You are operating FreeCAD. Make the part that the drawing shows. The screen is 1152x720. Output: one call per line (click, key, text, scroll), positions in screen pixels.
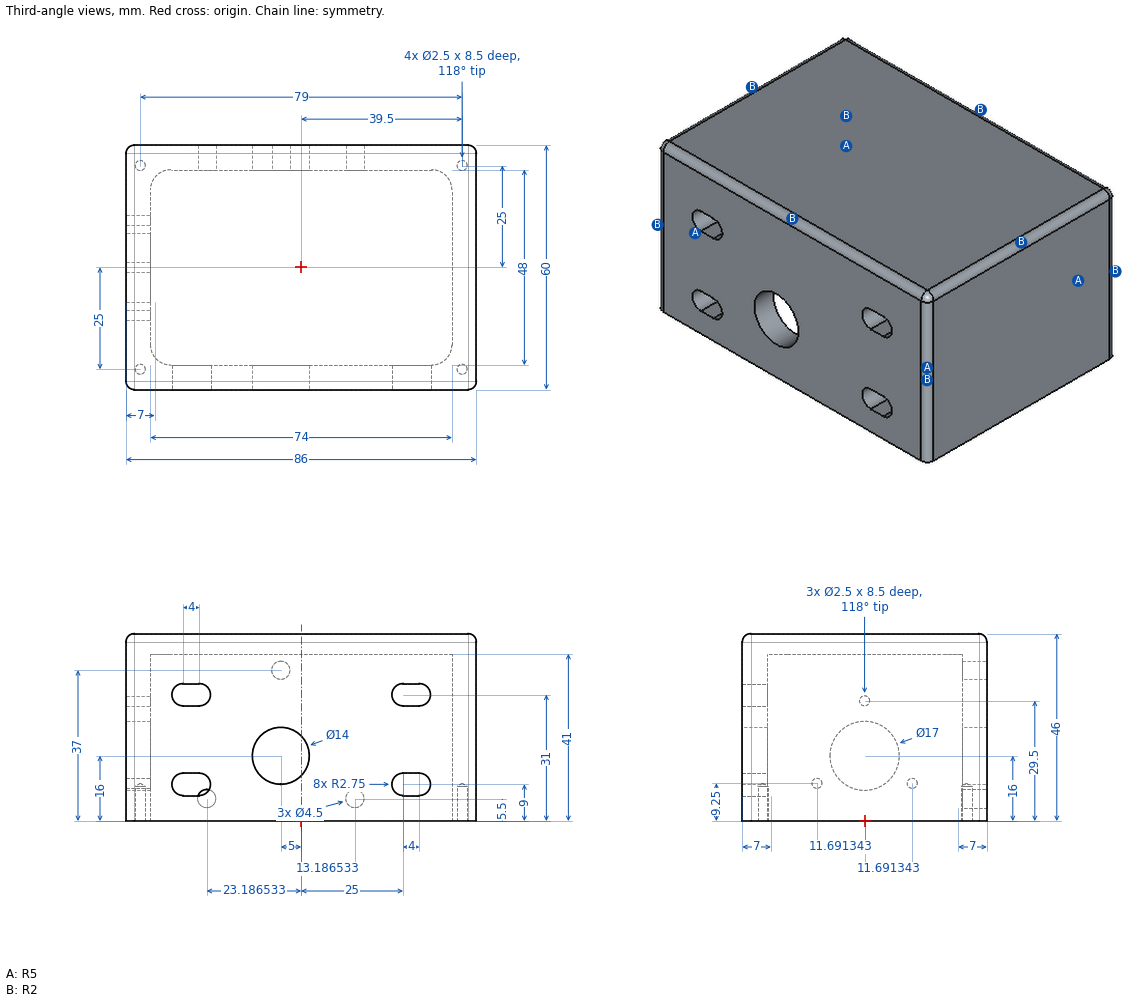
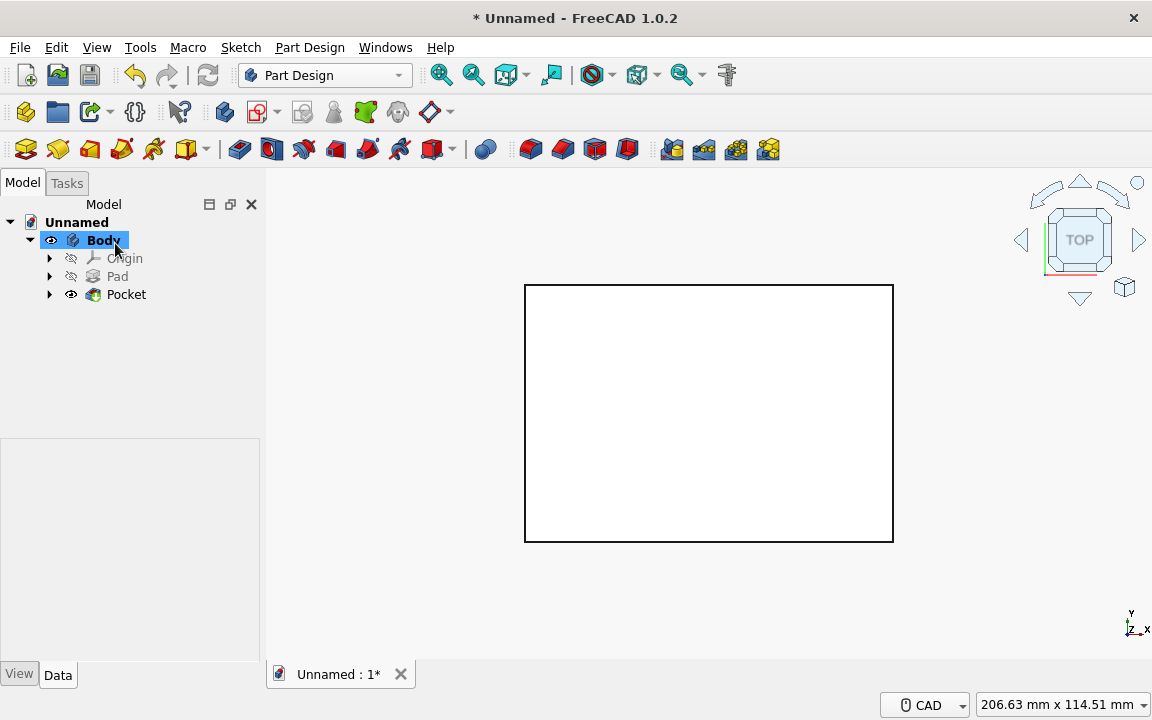
key(1)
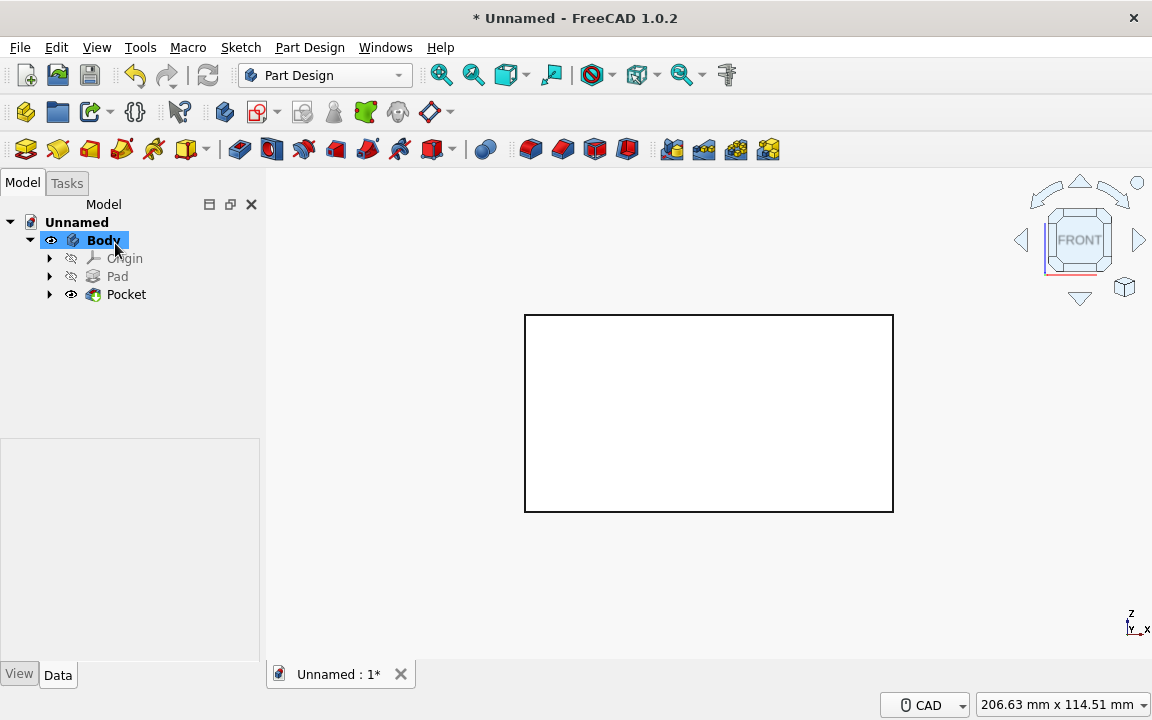
key(v)
key(f)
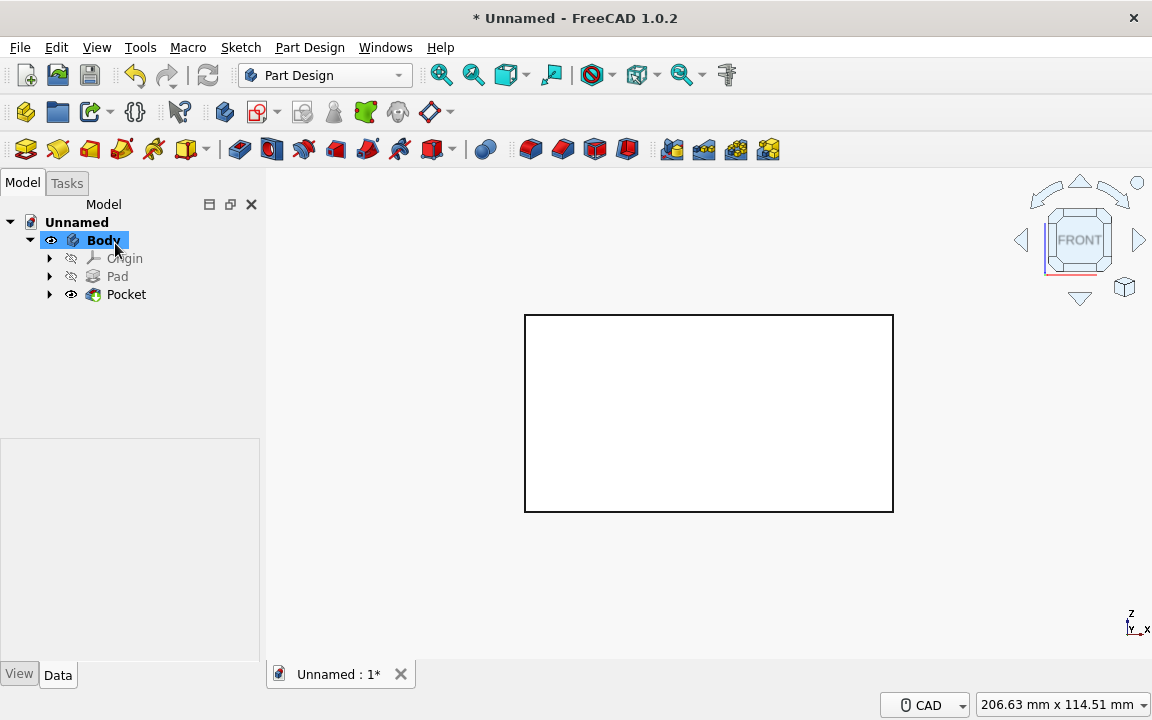
key(3)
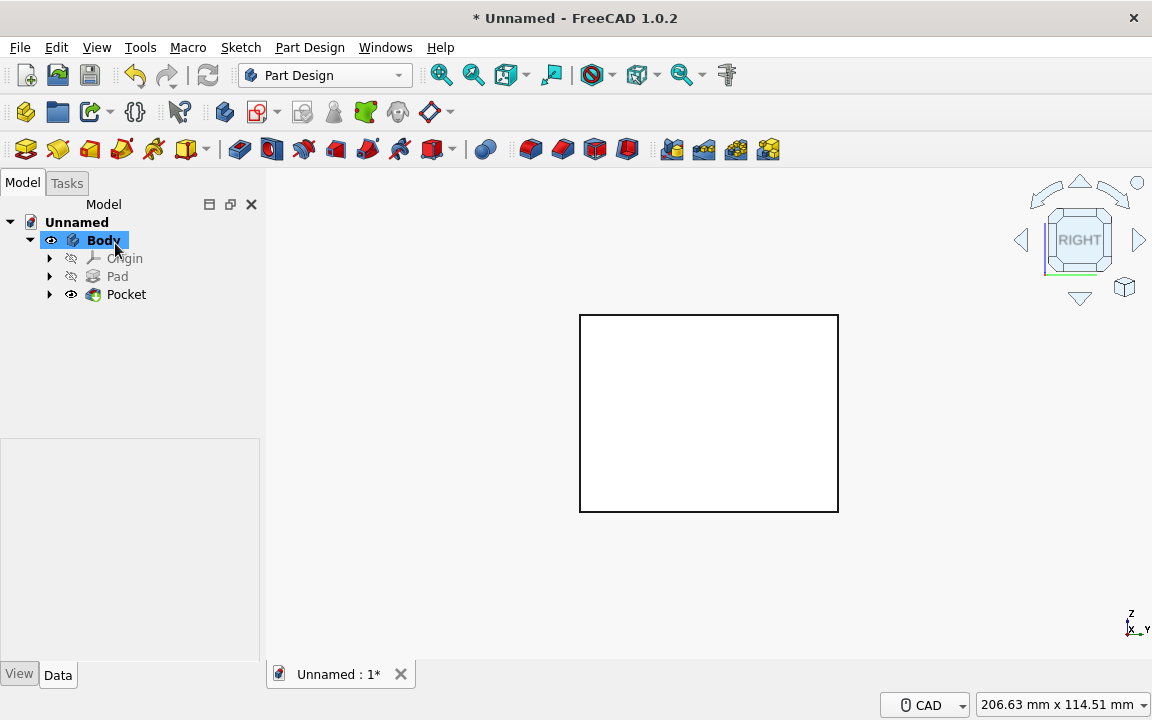
key(v)
key(f)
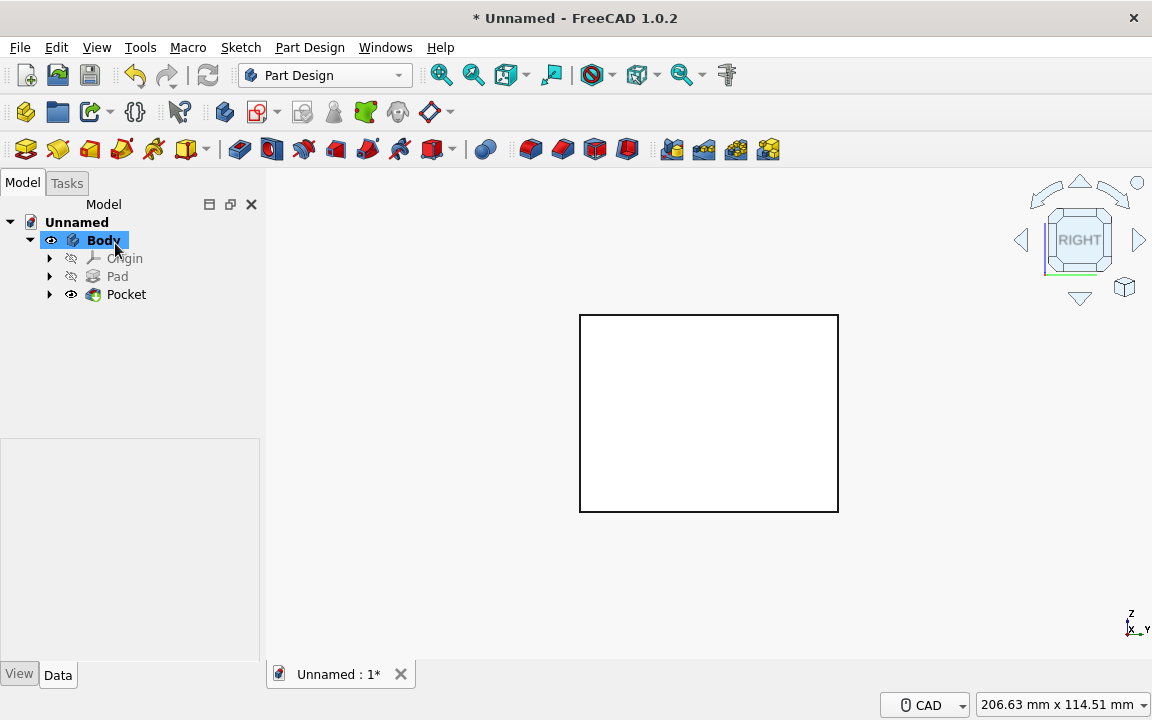
key(5)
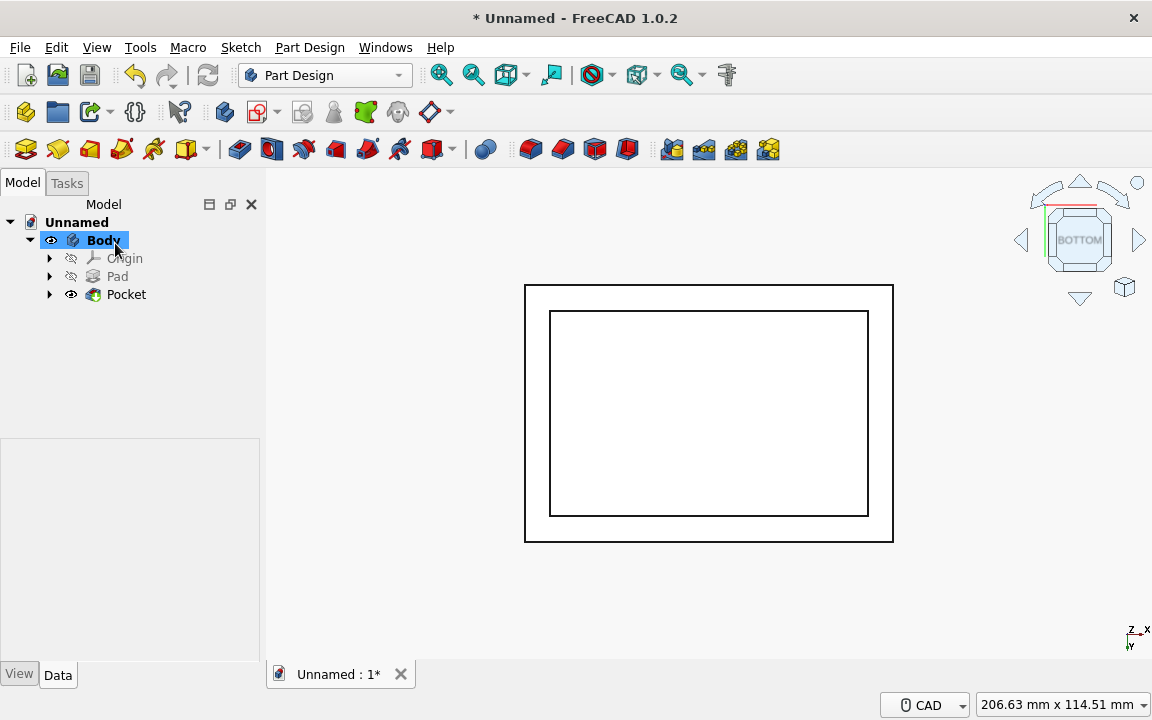
key(4)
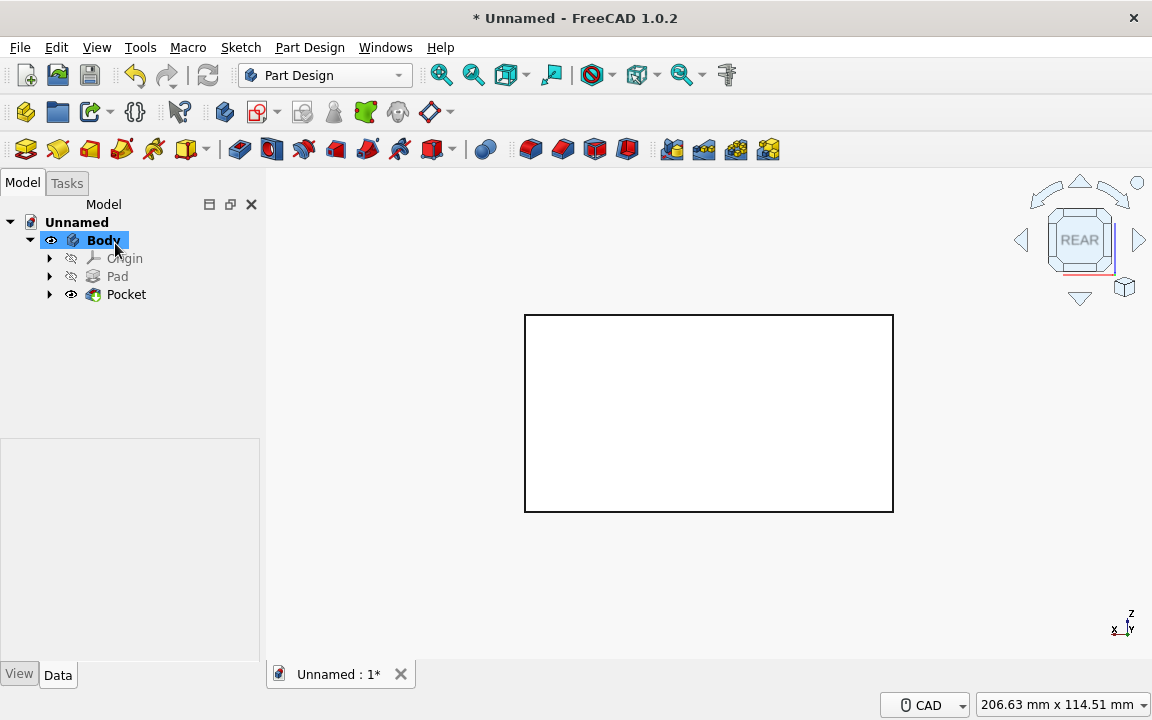
click(442, 76)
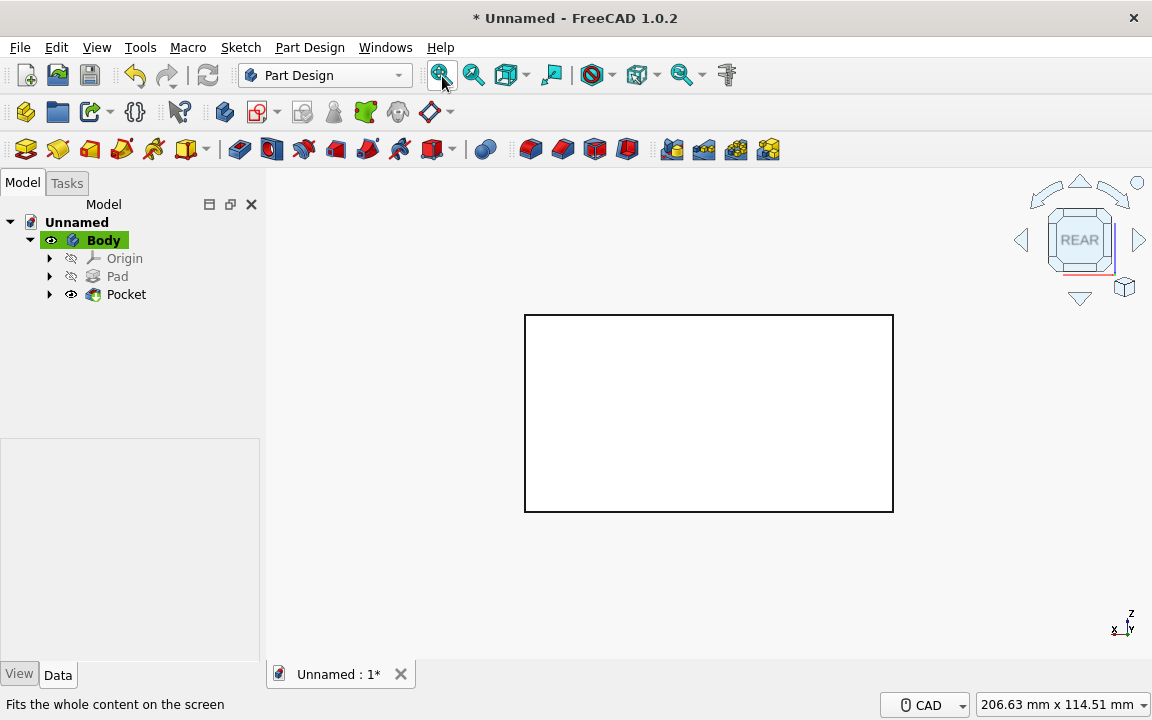
key(6)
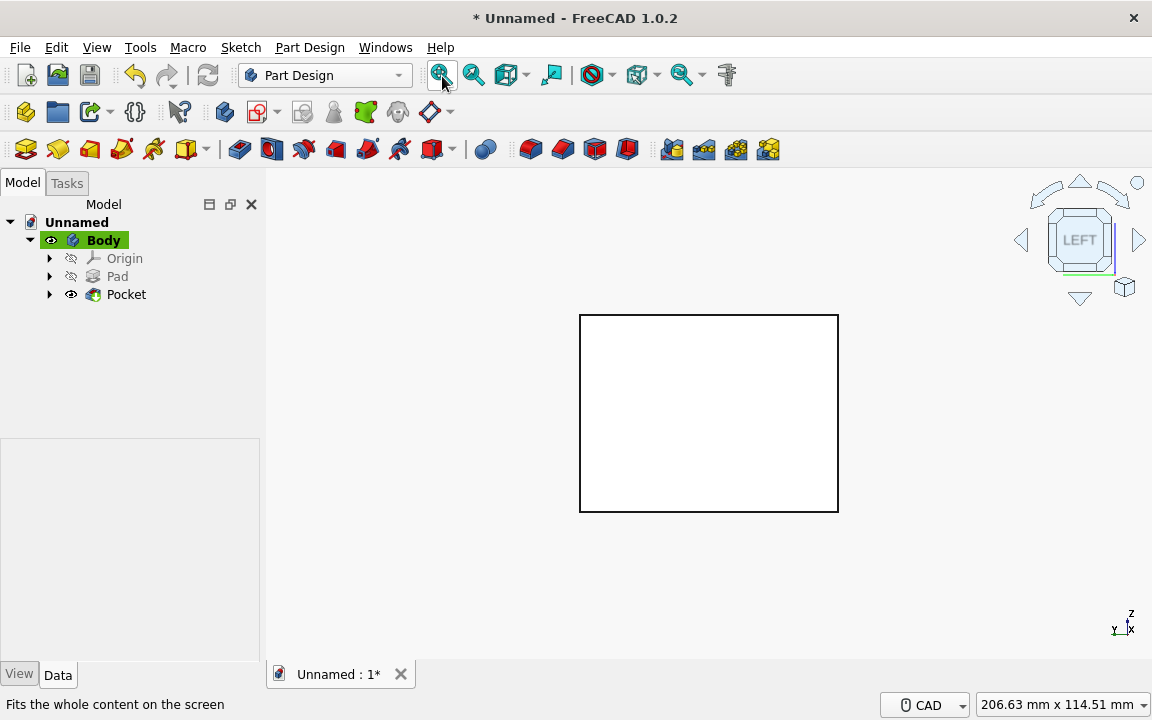
key(v)
key(f)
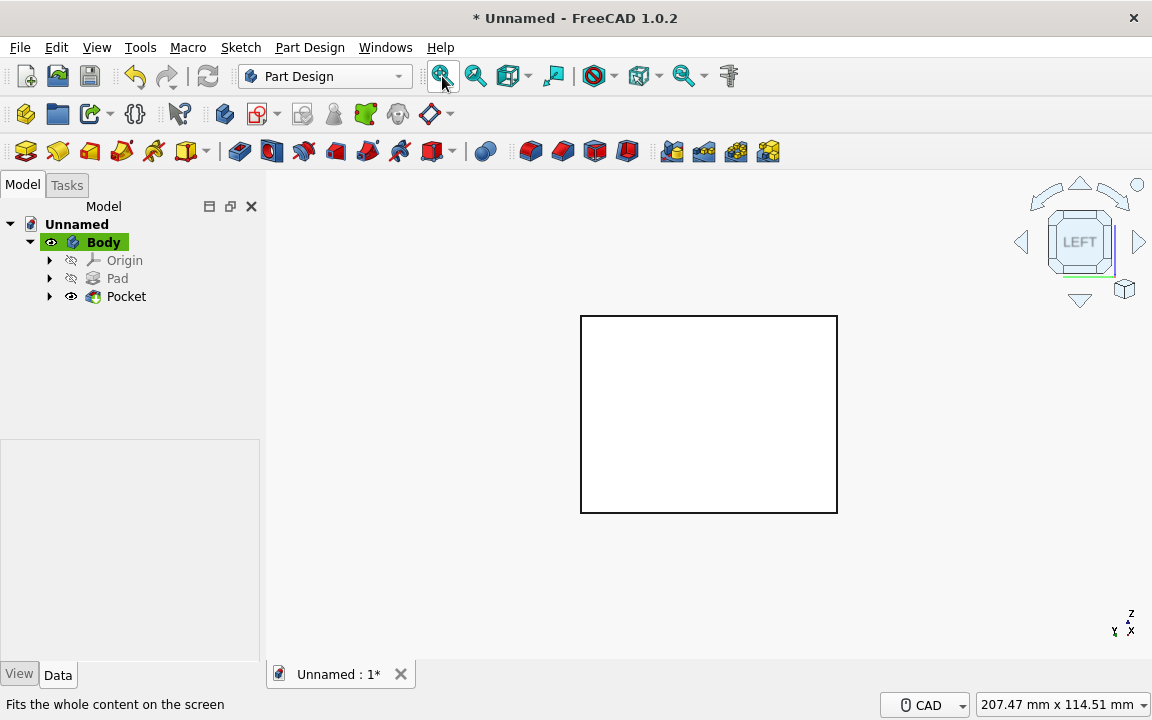
key(v)
key(3)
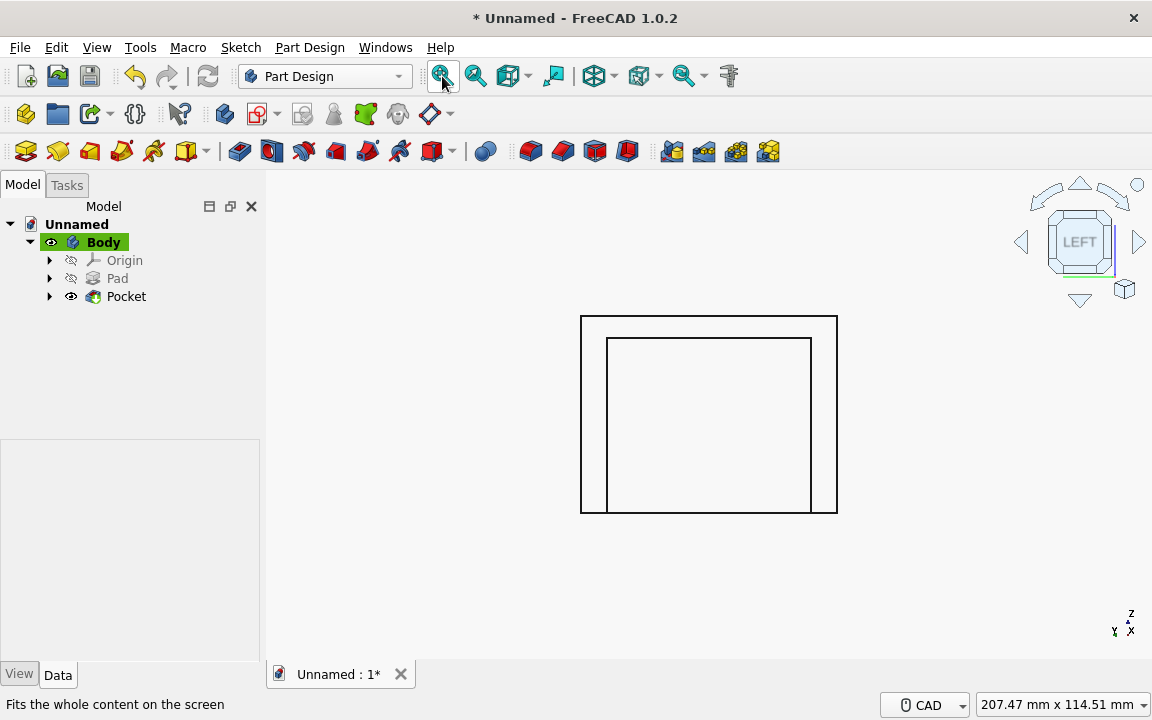
key(0)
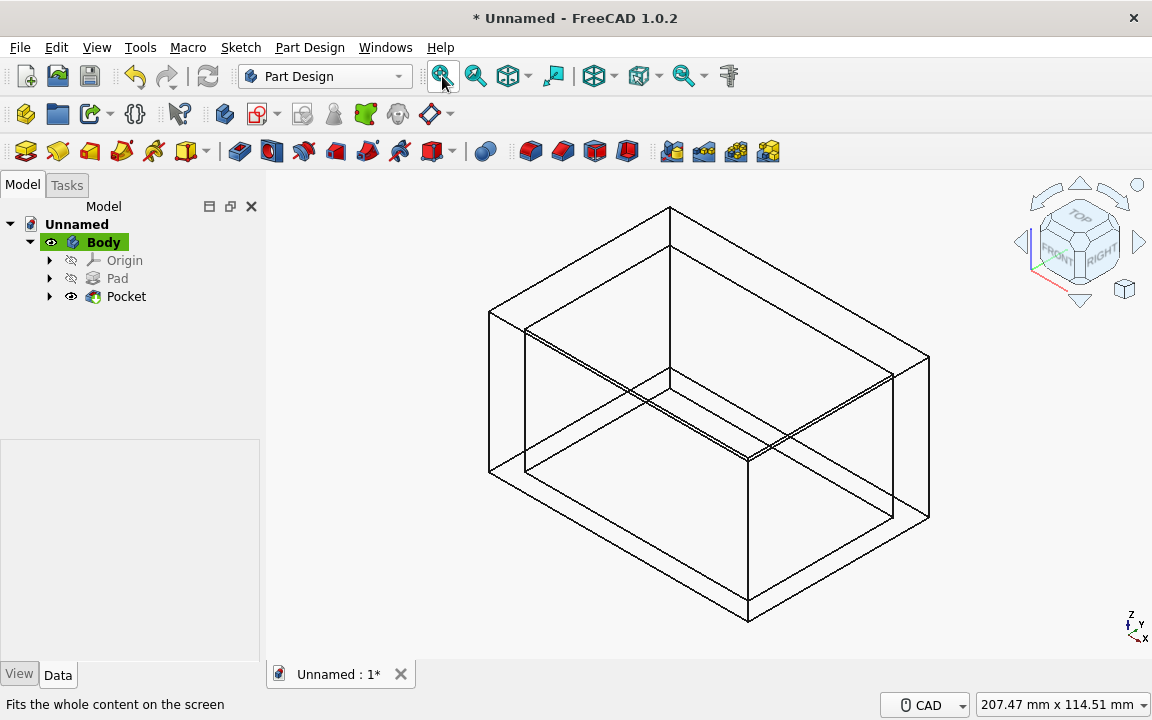
click(525, 400)